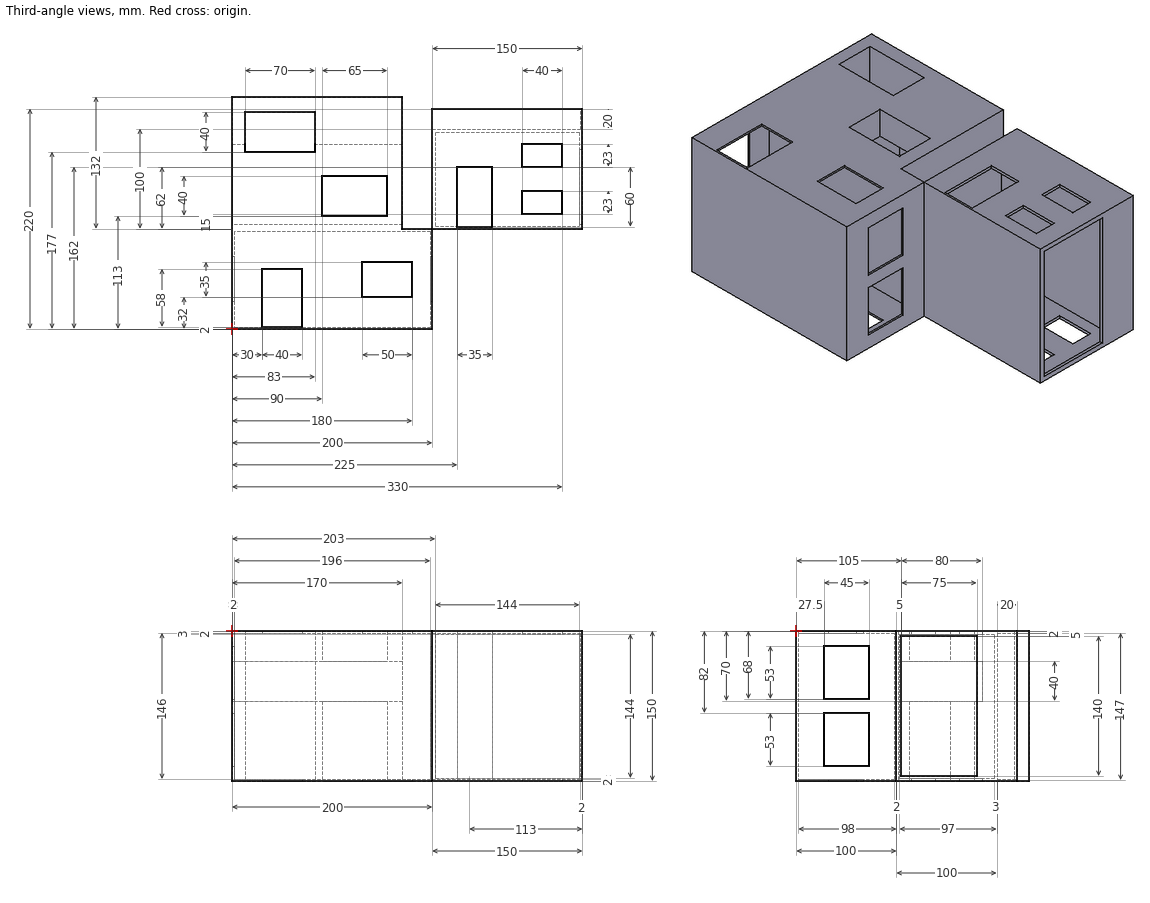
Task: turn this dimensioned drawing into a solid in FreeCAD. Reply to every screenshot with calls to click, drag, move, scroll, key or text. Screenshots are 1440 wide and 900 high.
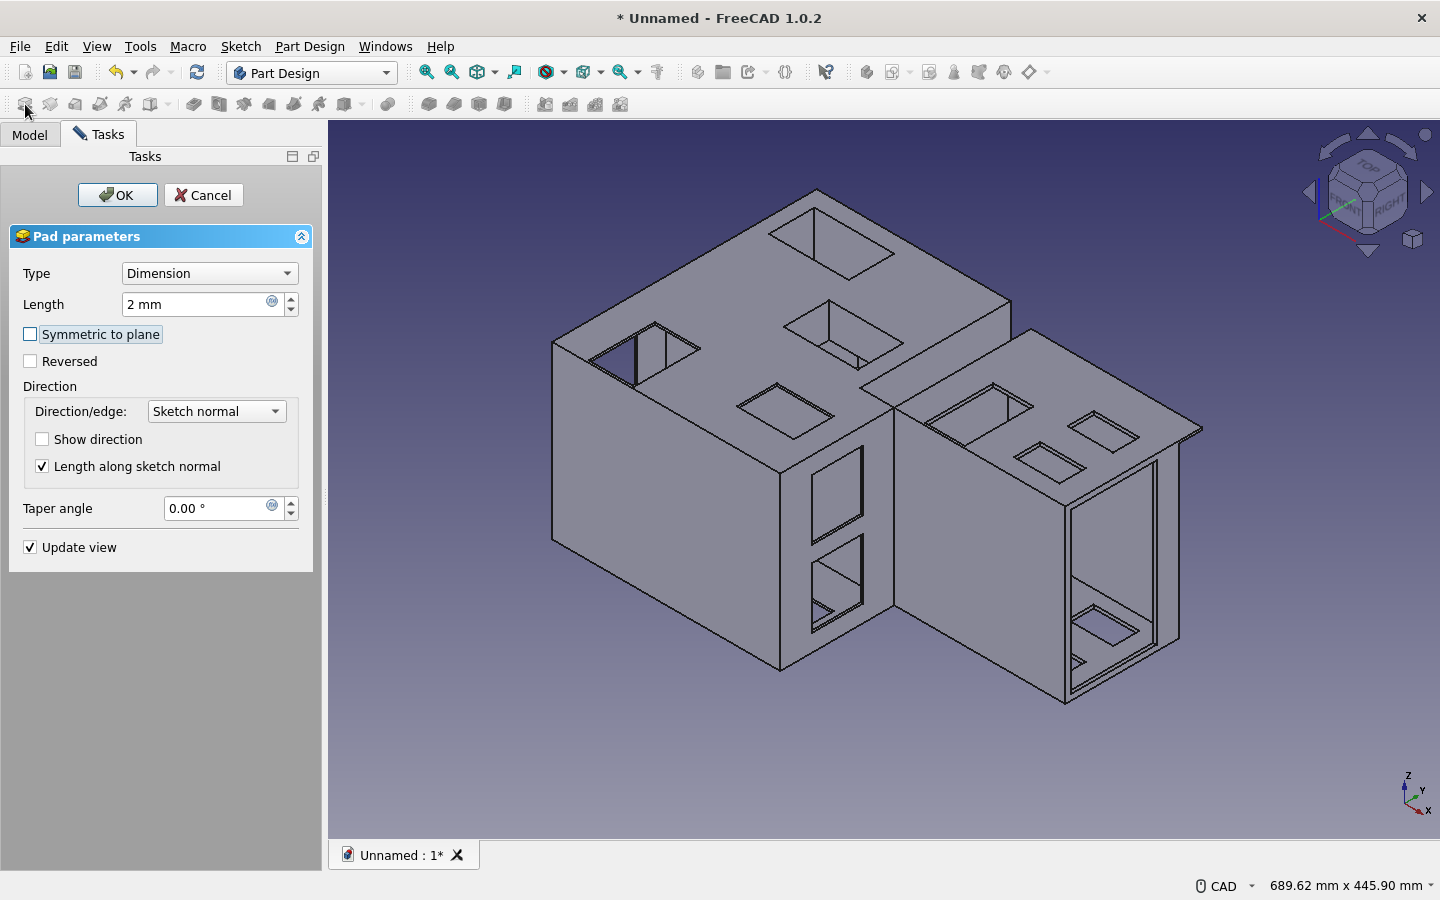
click(31, 361)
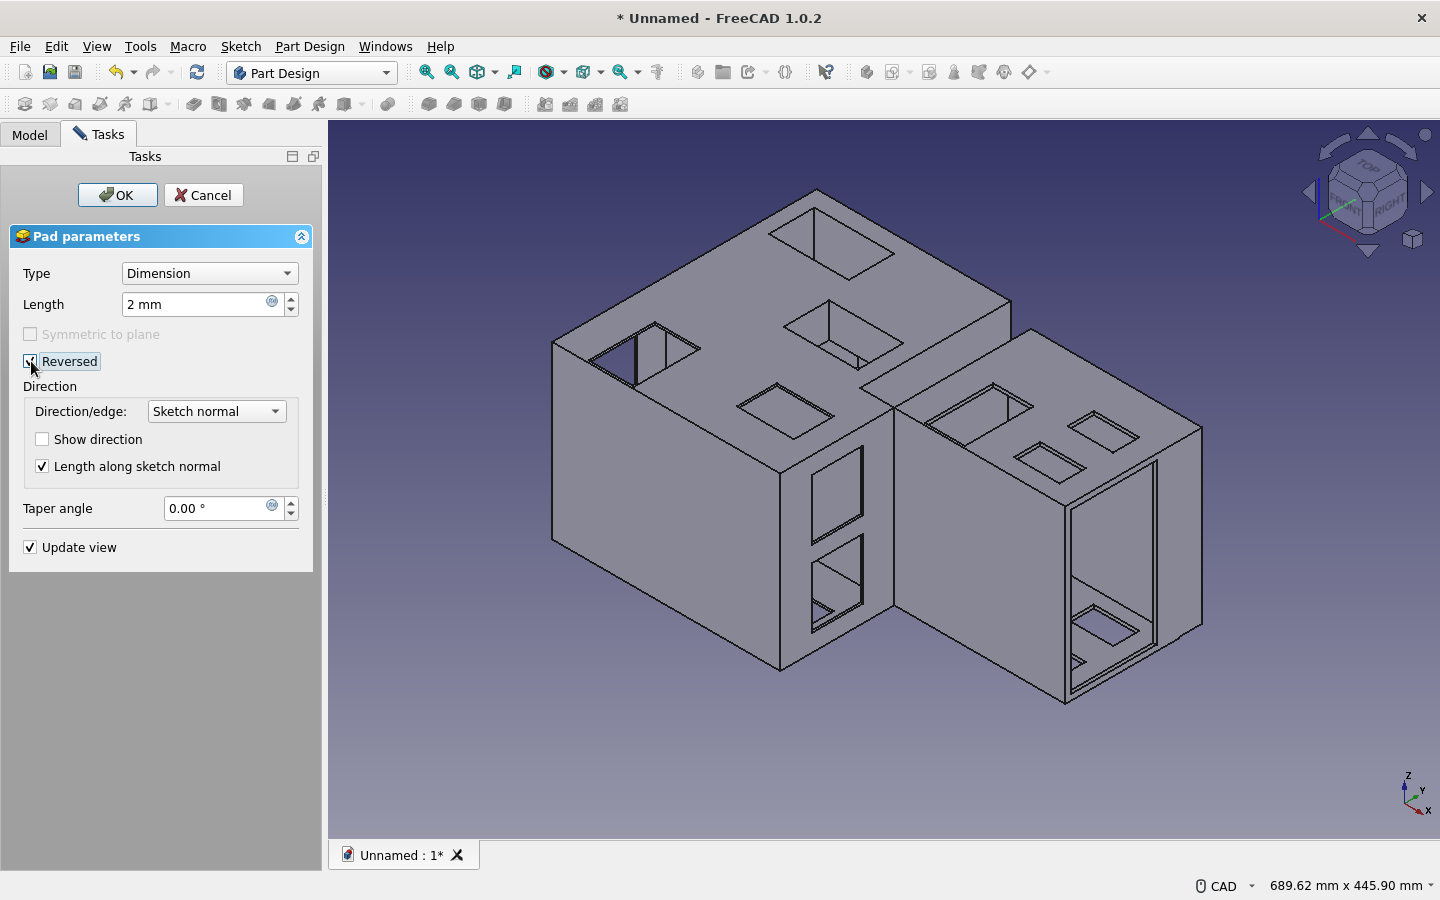
click(118, 195)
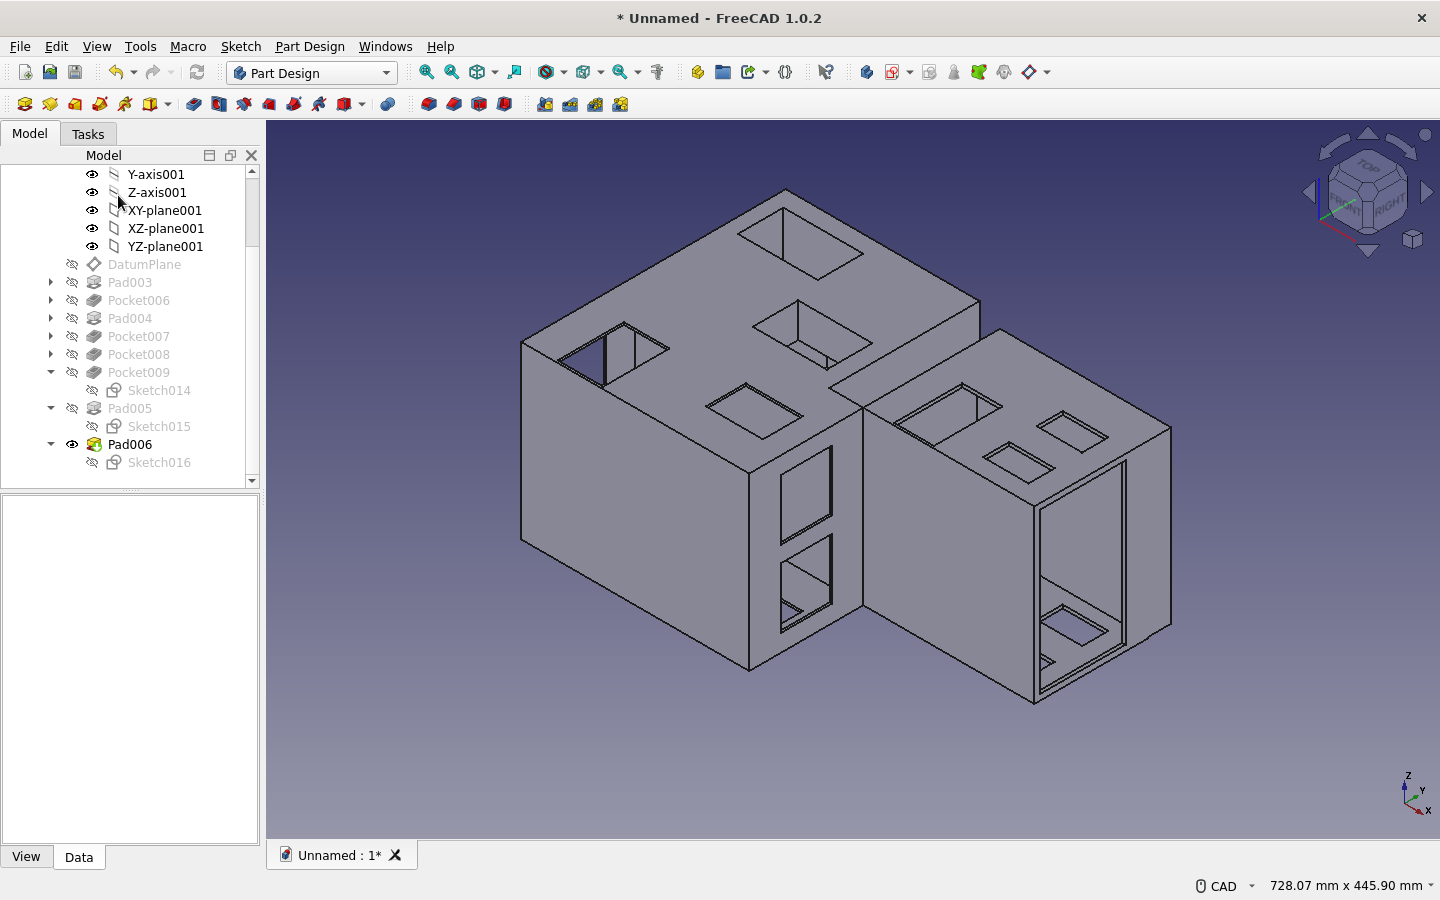
key(5)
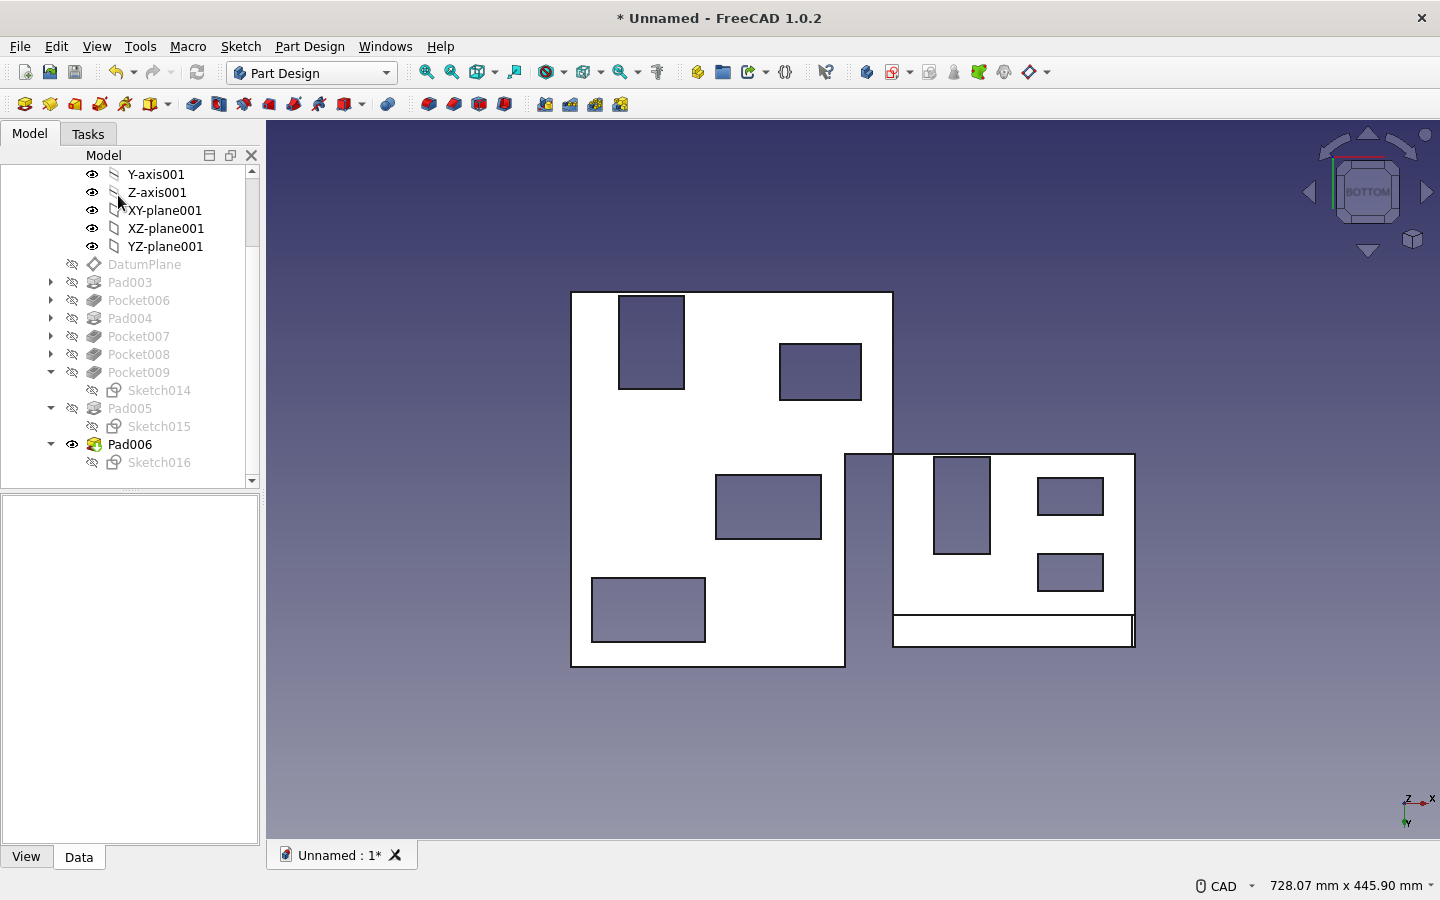
click(427, 72)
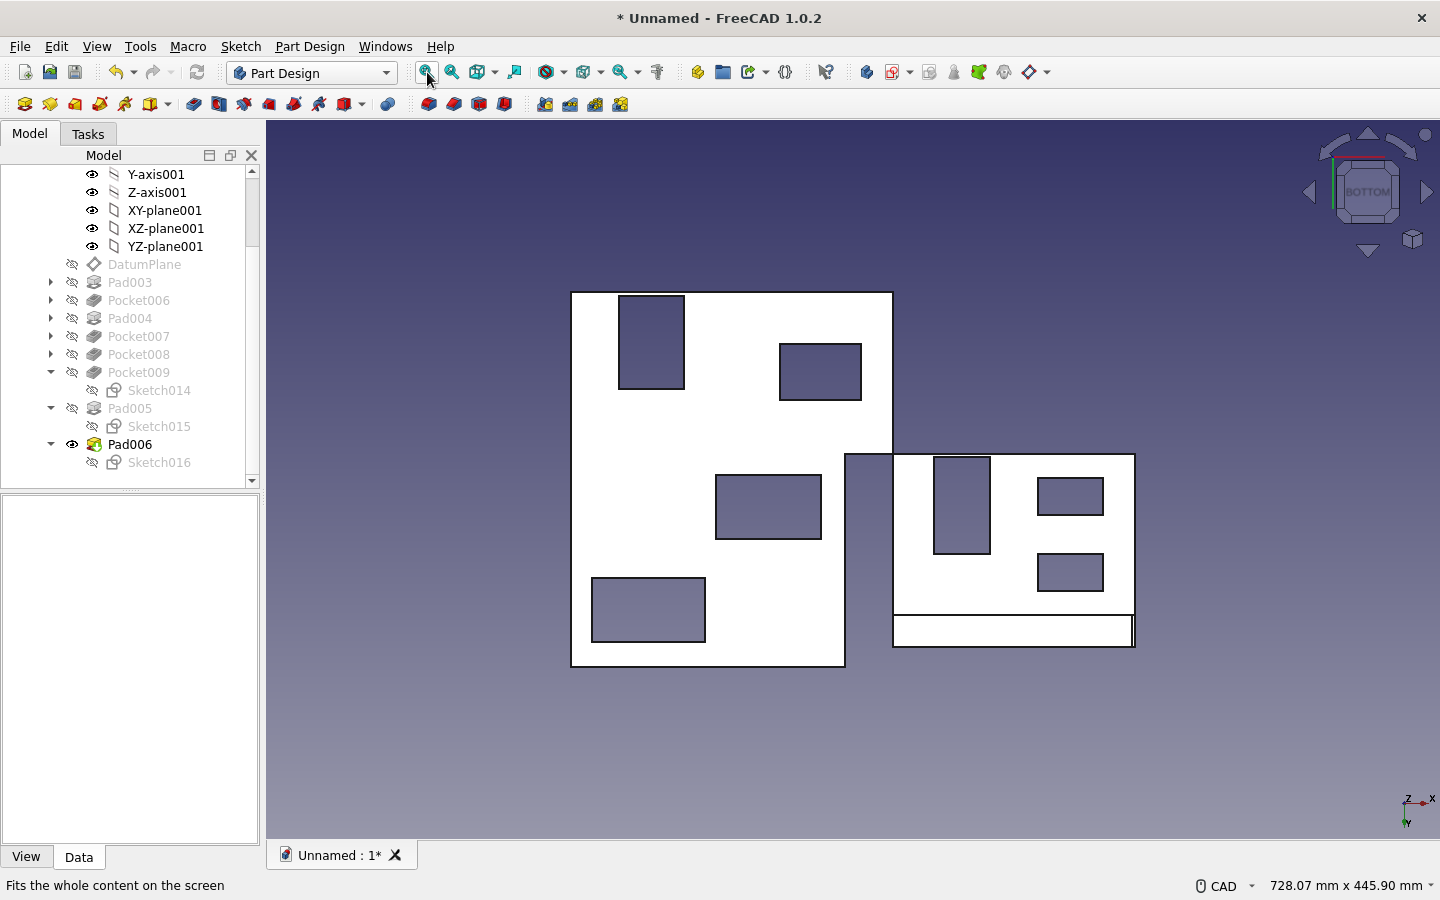
click(980, 579)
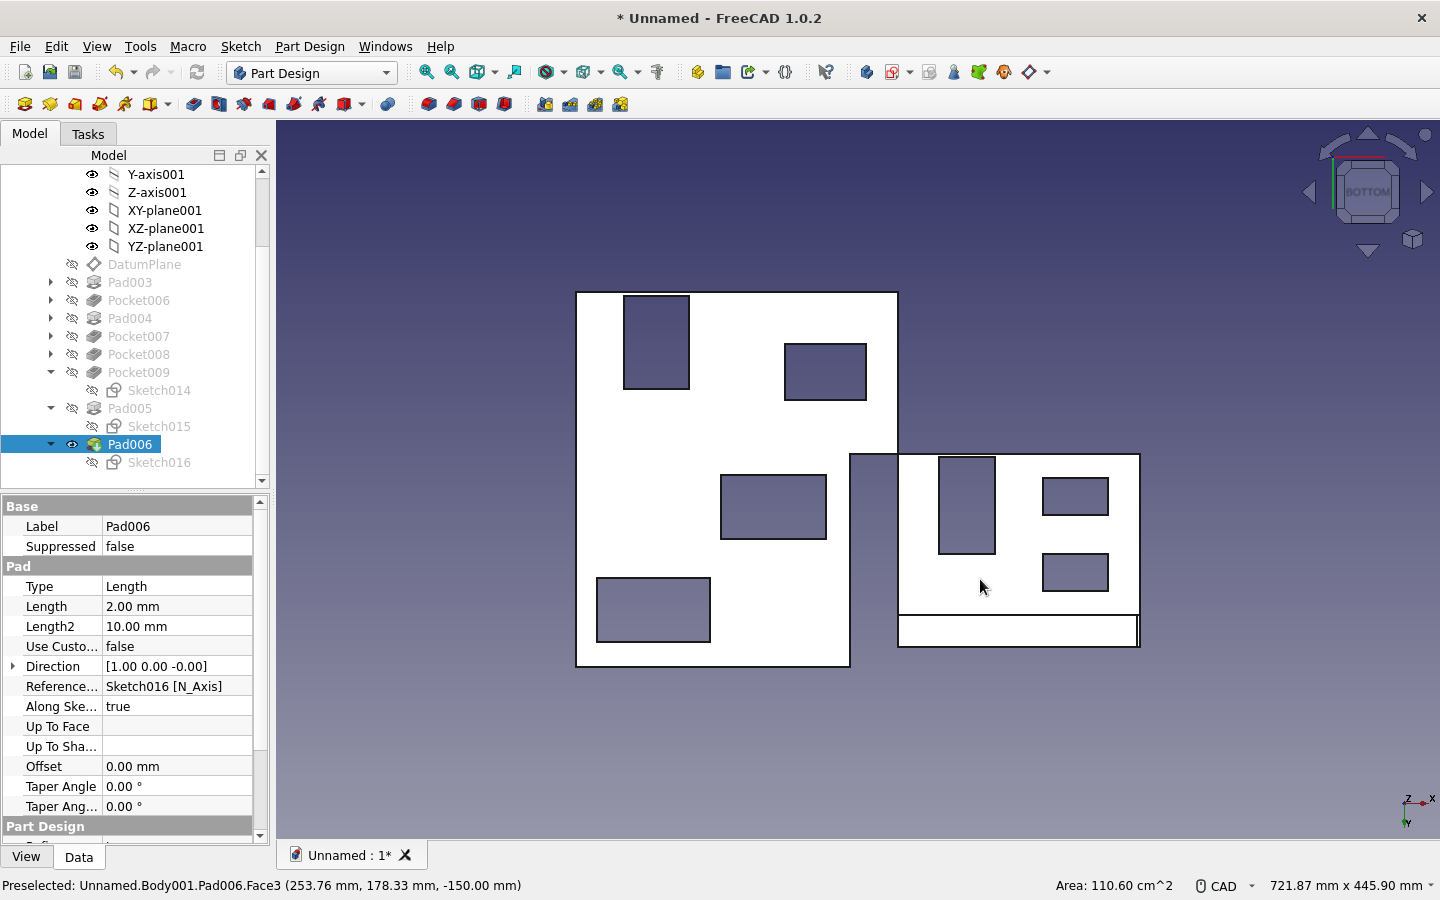
click(892, 72)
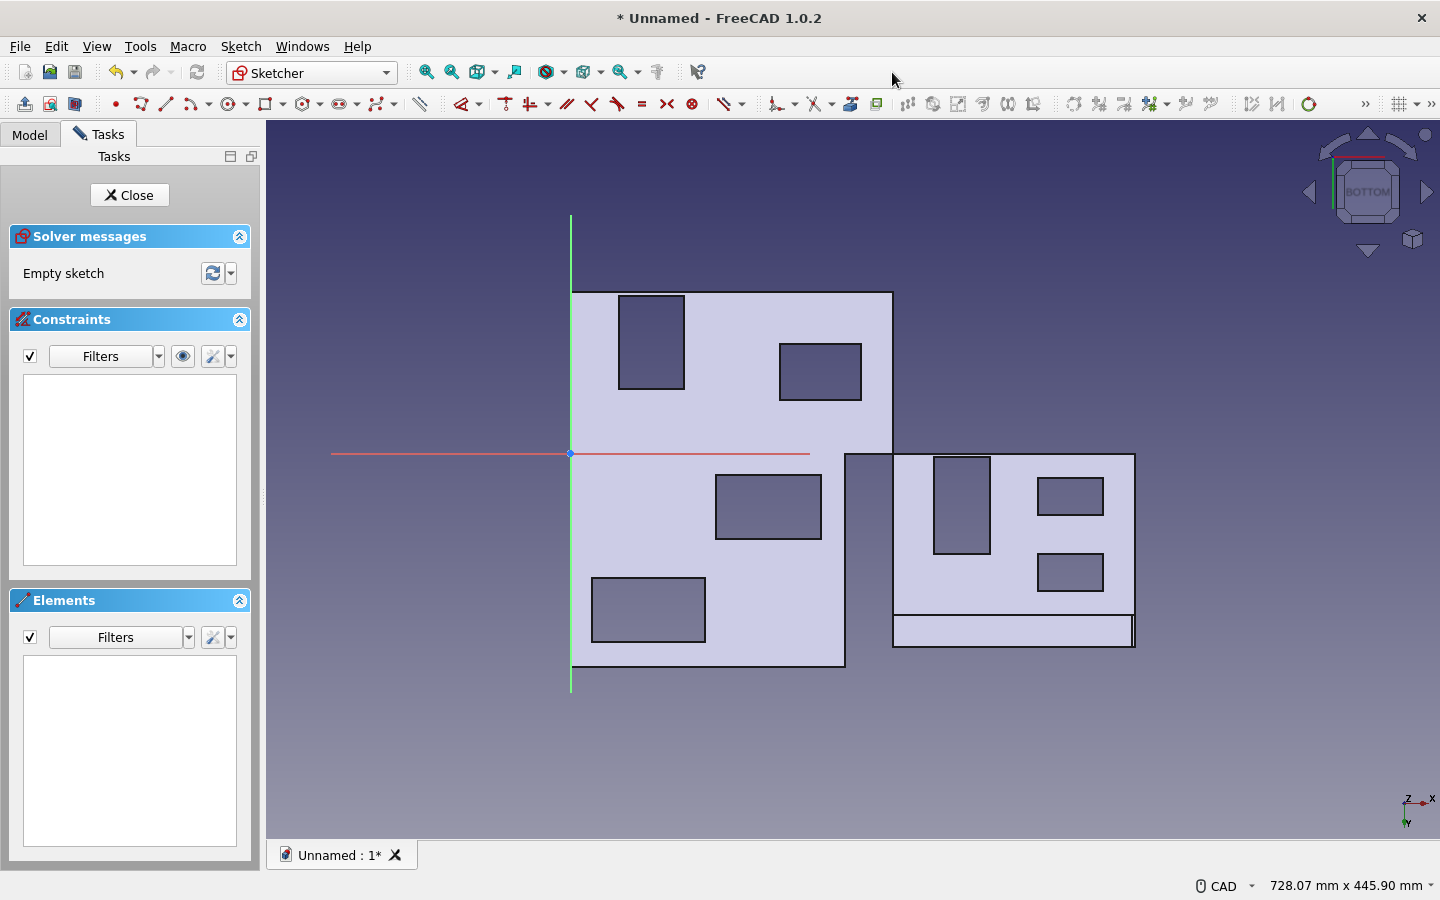
click(264, 104)